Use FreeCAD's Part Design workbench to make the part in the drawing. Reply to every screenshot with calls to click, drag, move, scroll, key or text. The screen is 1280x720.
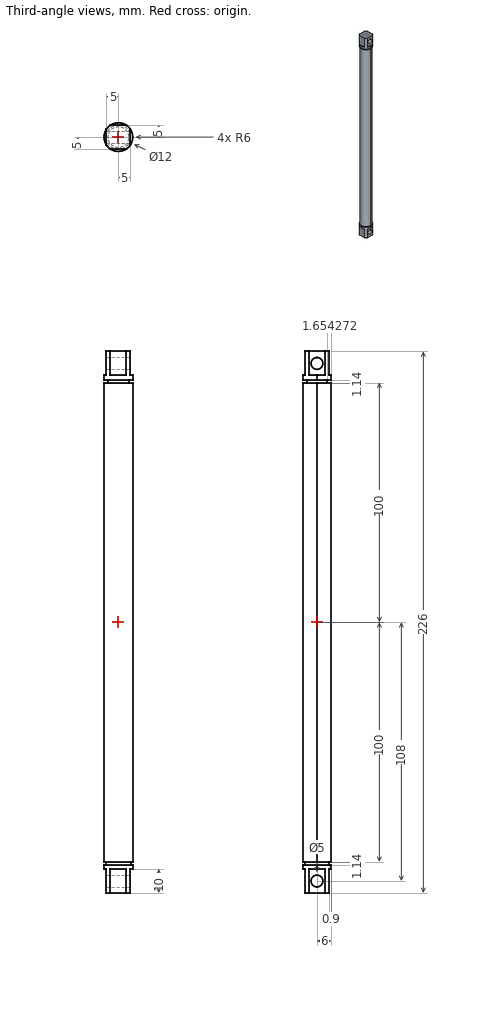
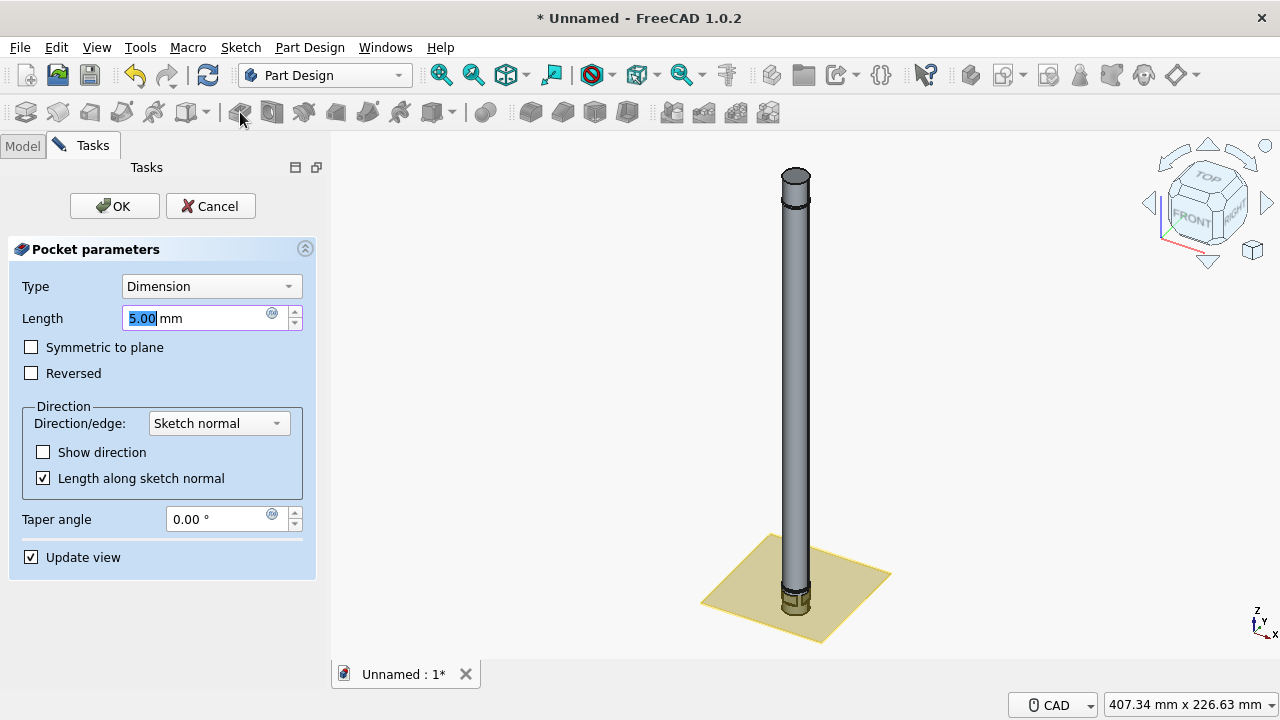
text(10)
key(Tab)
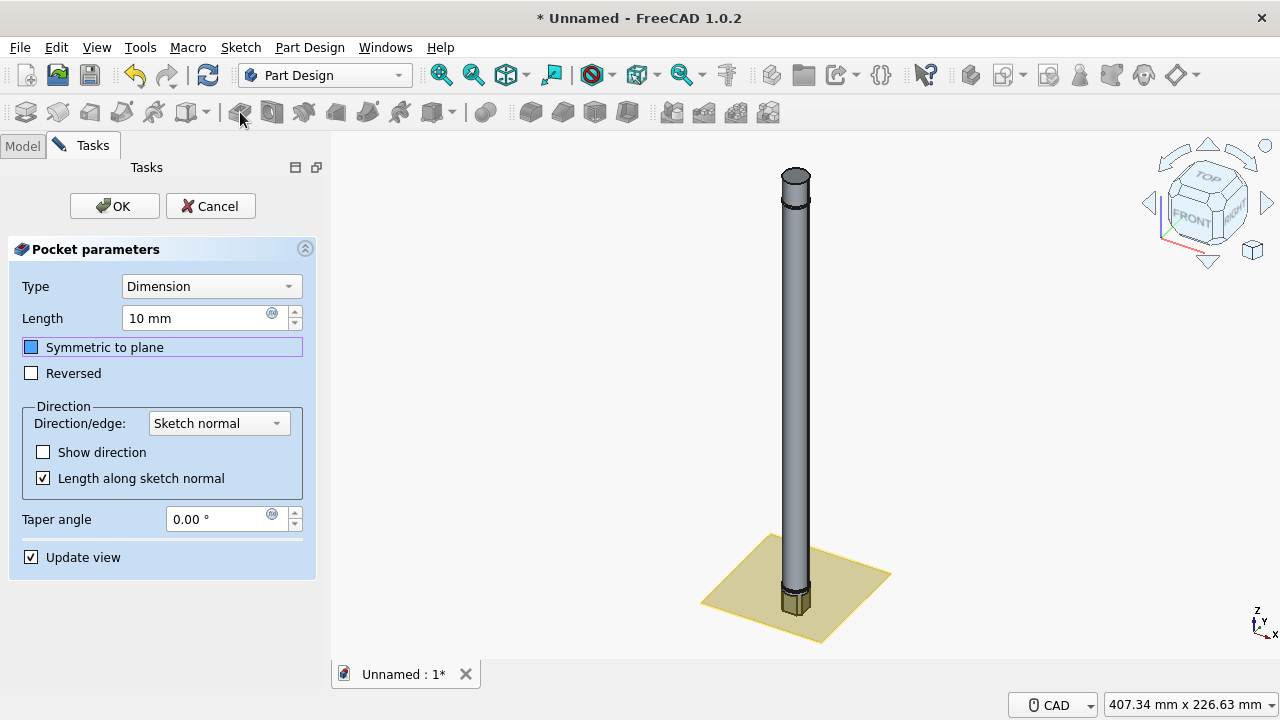
click(115, 206)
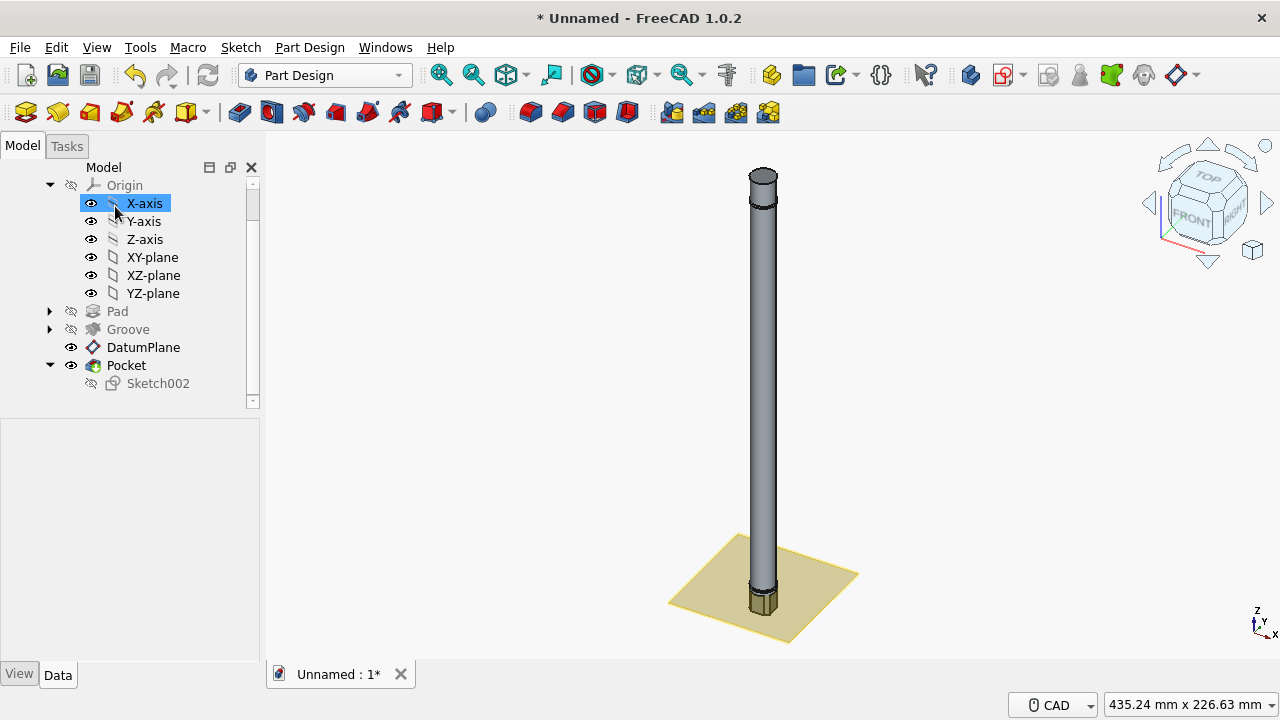
click(116, 347)
key(space)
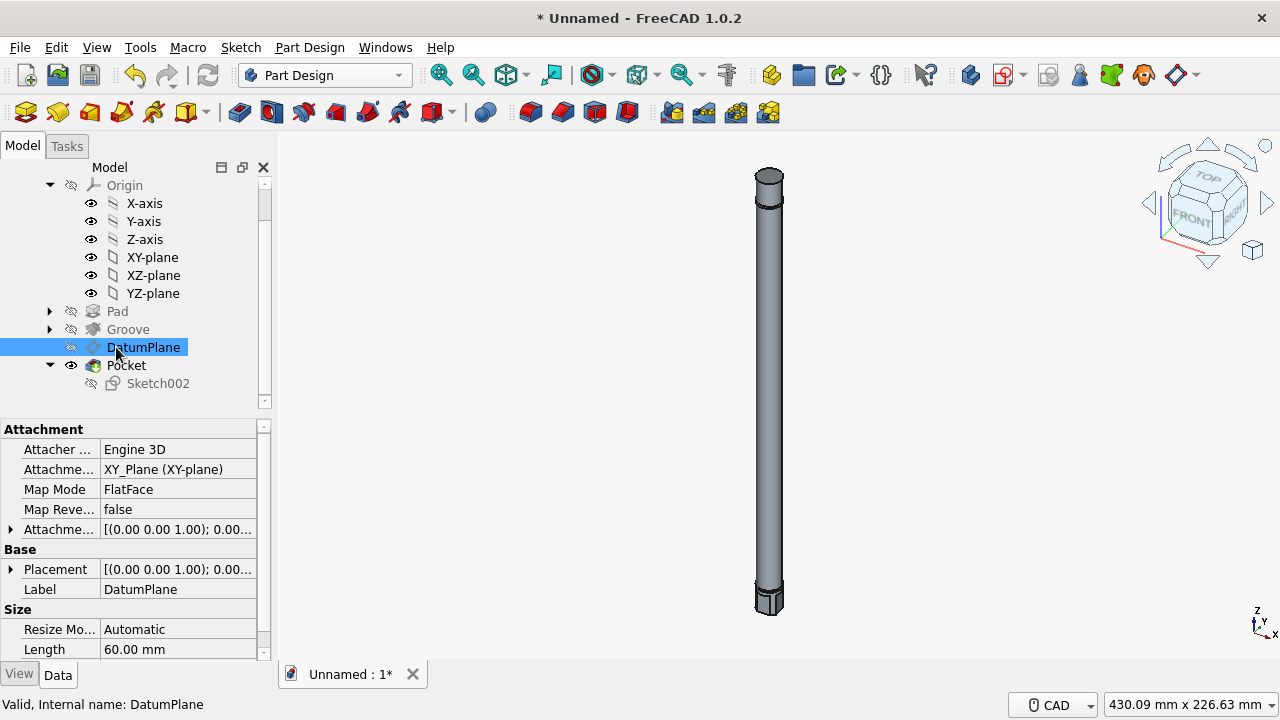
key(6)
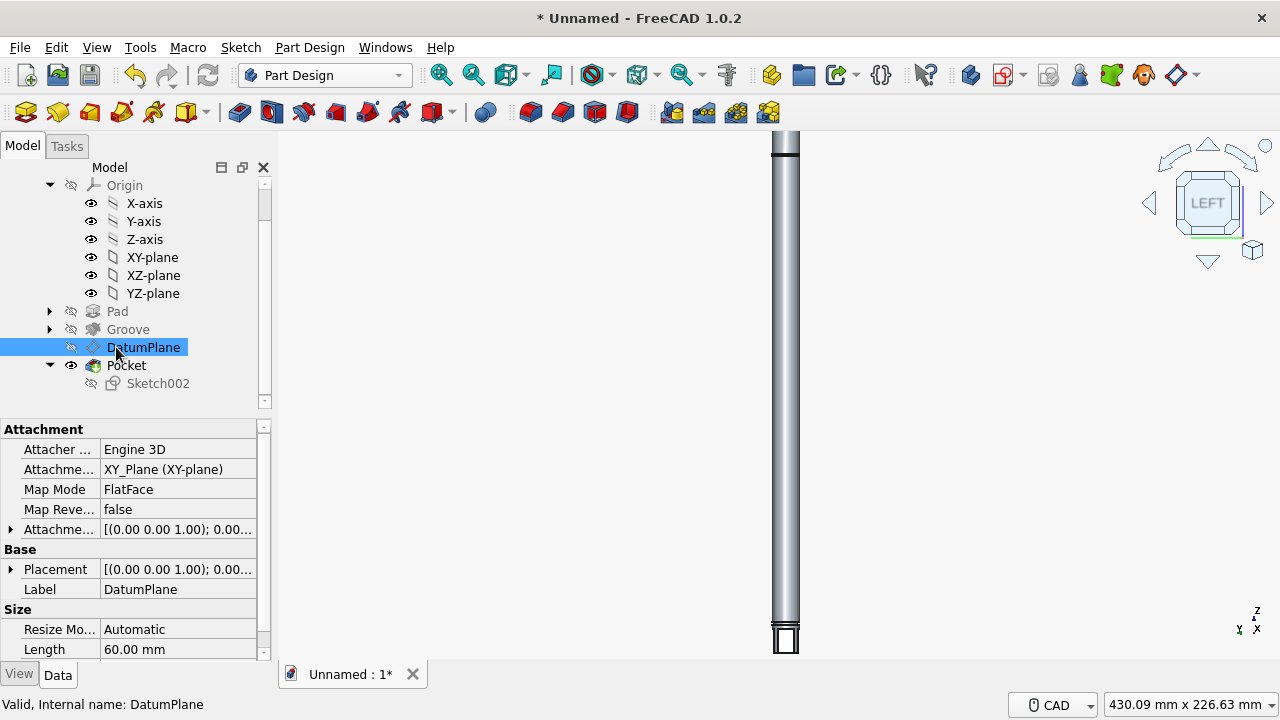
click(442, 76)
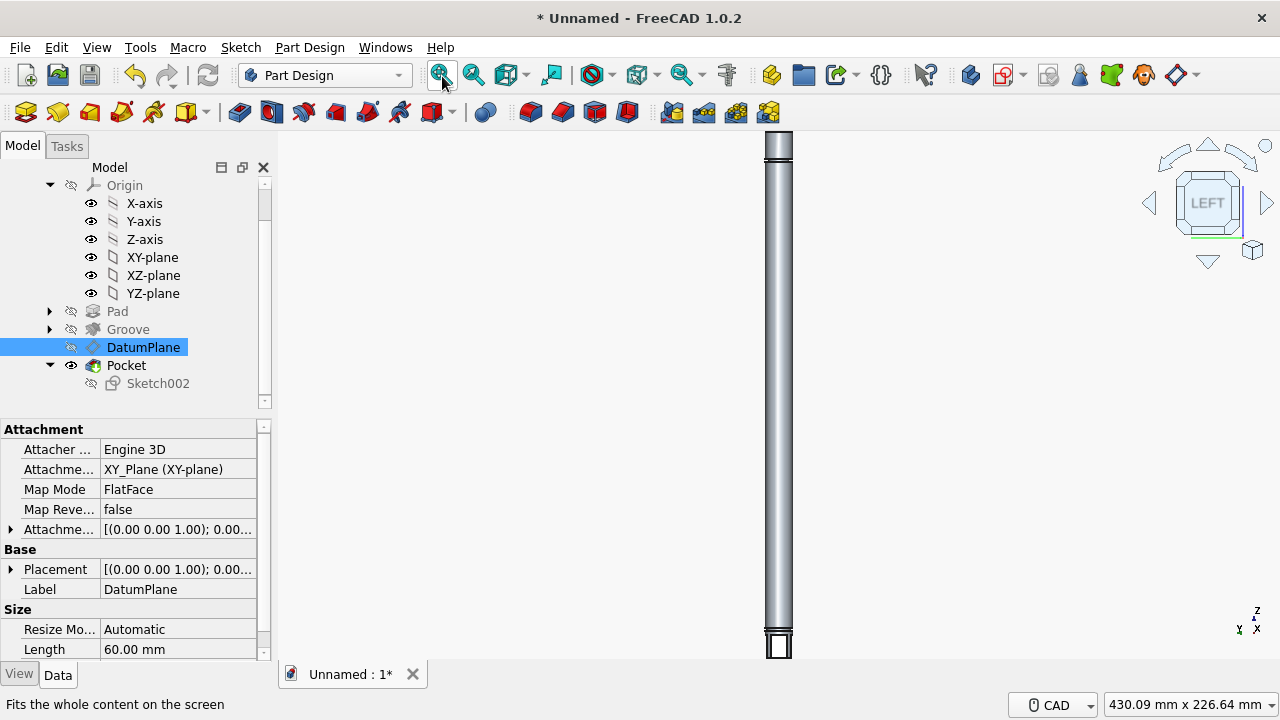
key(2)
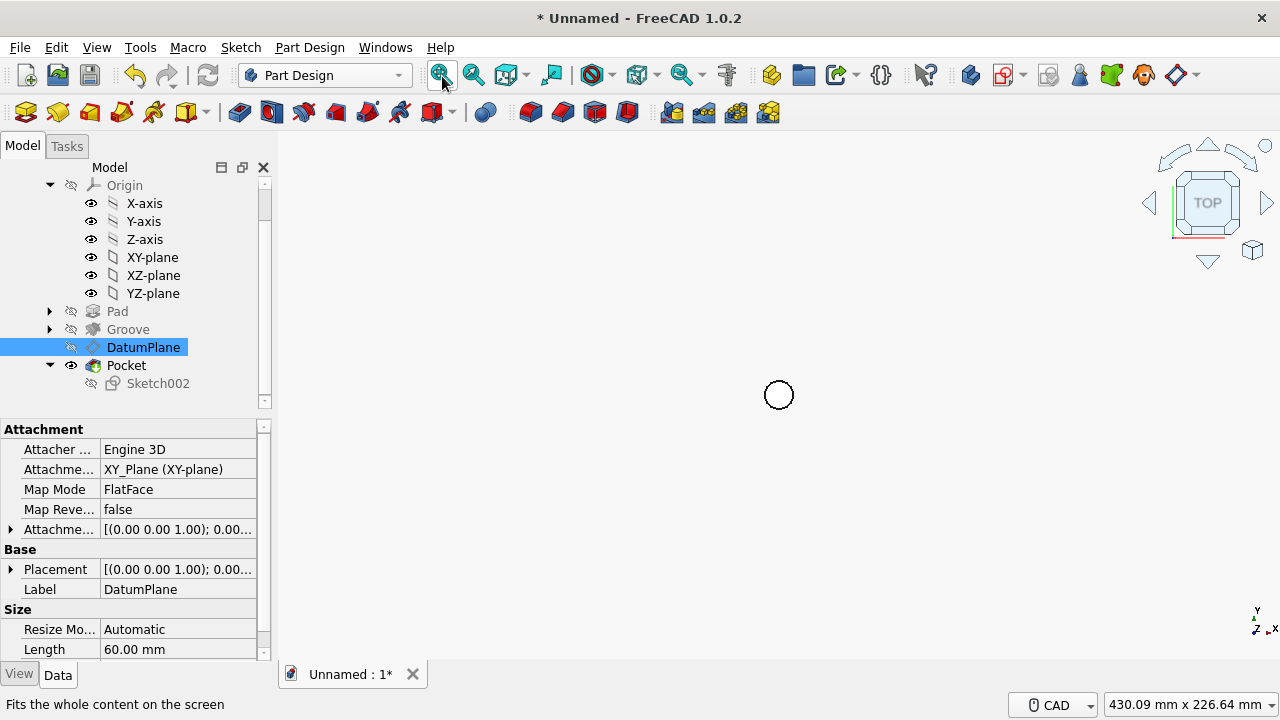
click(442, 76)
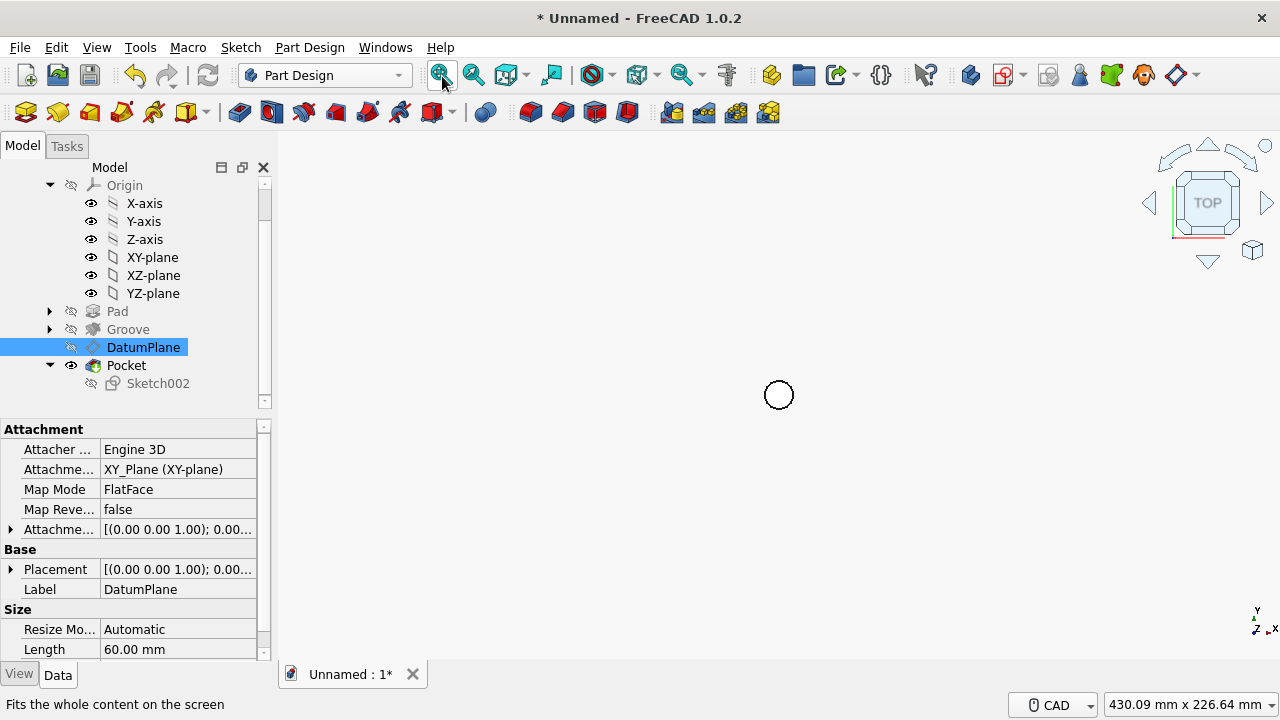
key(1)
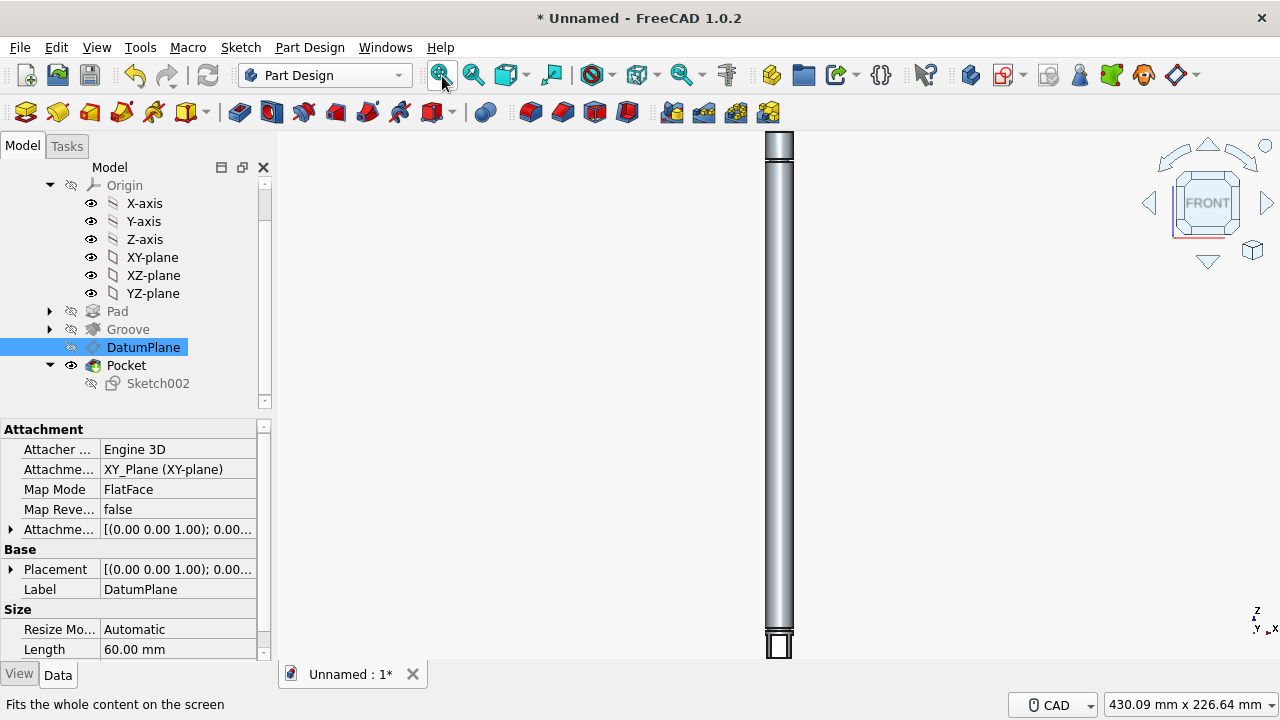
click(136, 293)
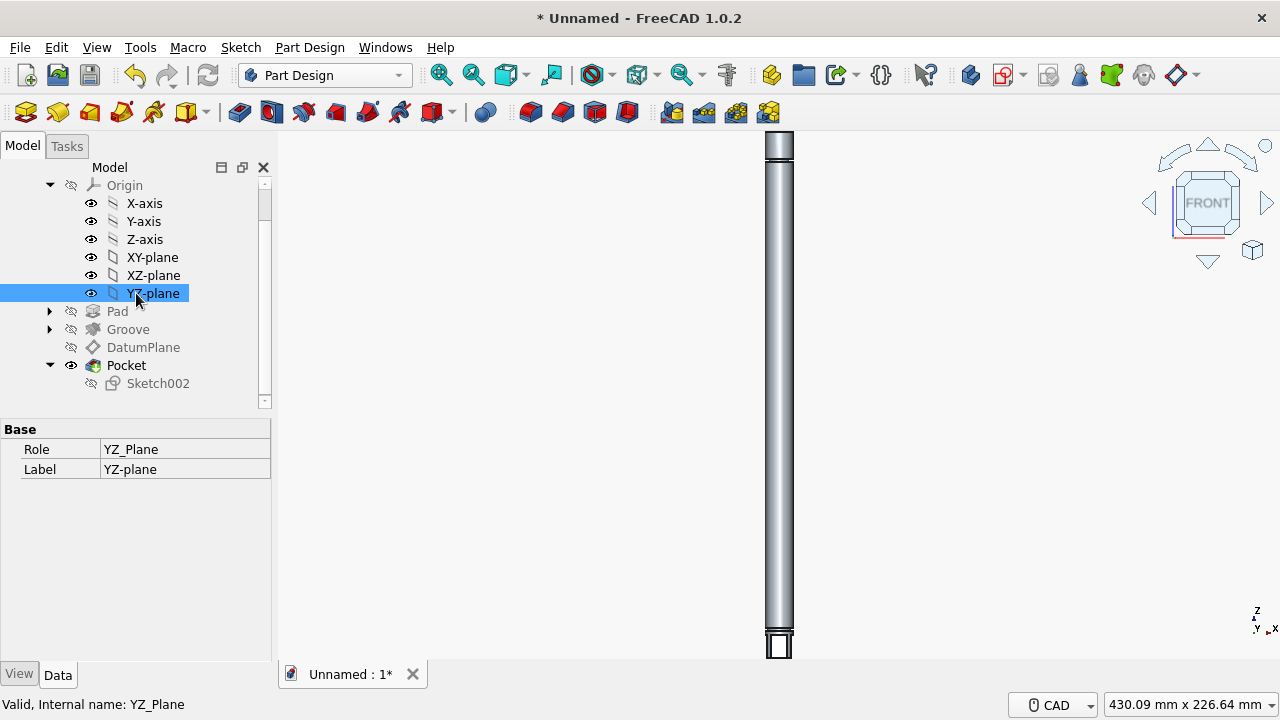
click(1176, 76)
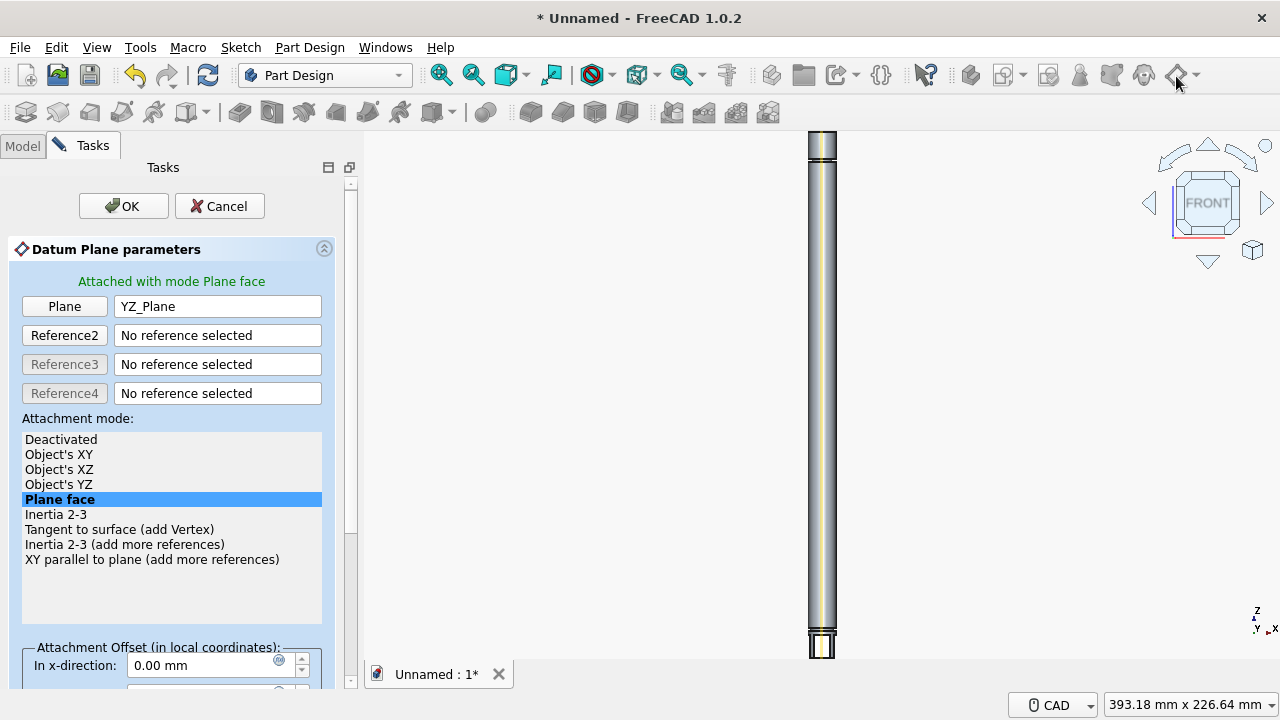
scroll(351, 432, down, 2)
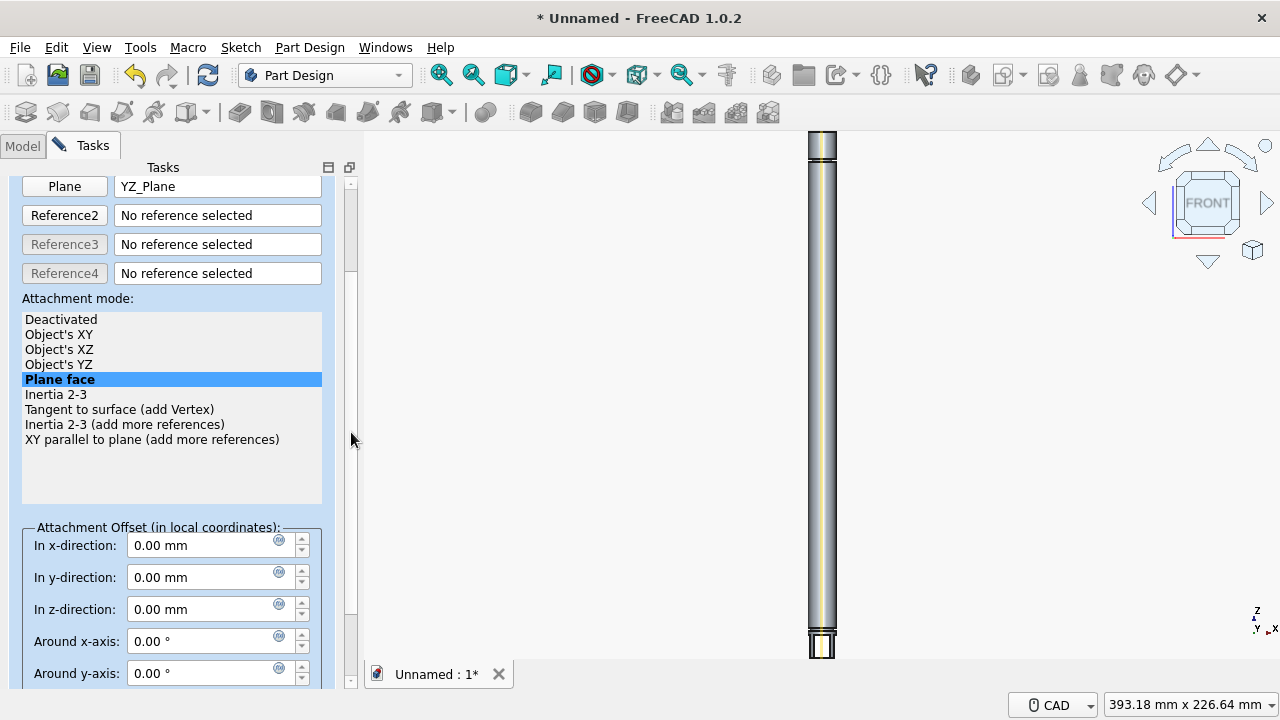
triple_click(210, 609)